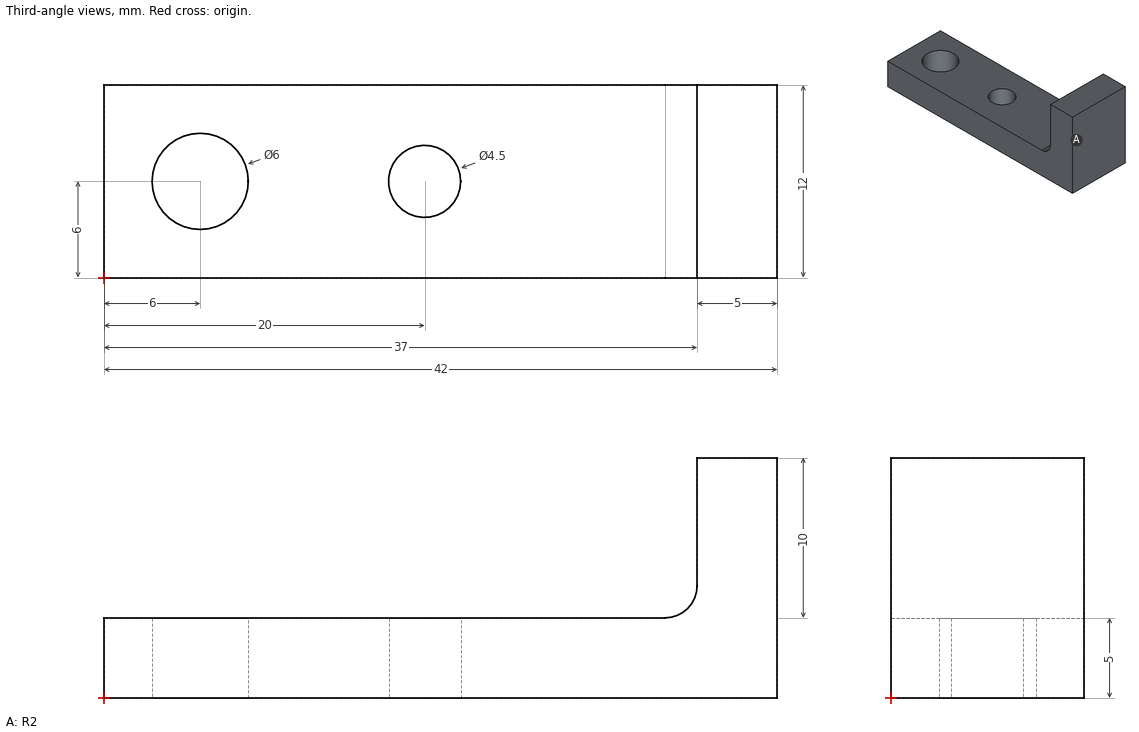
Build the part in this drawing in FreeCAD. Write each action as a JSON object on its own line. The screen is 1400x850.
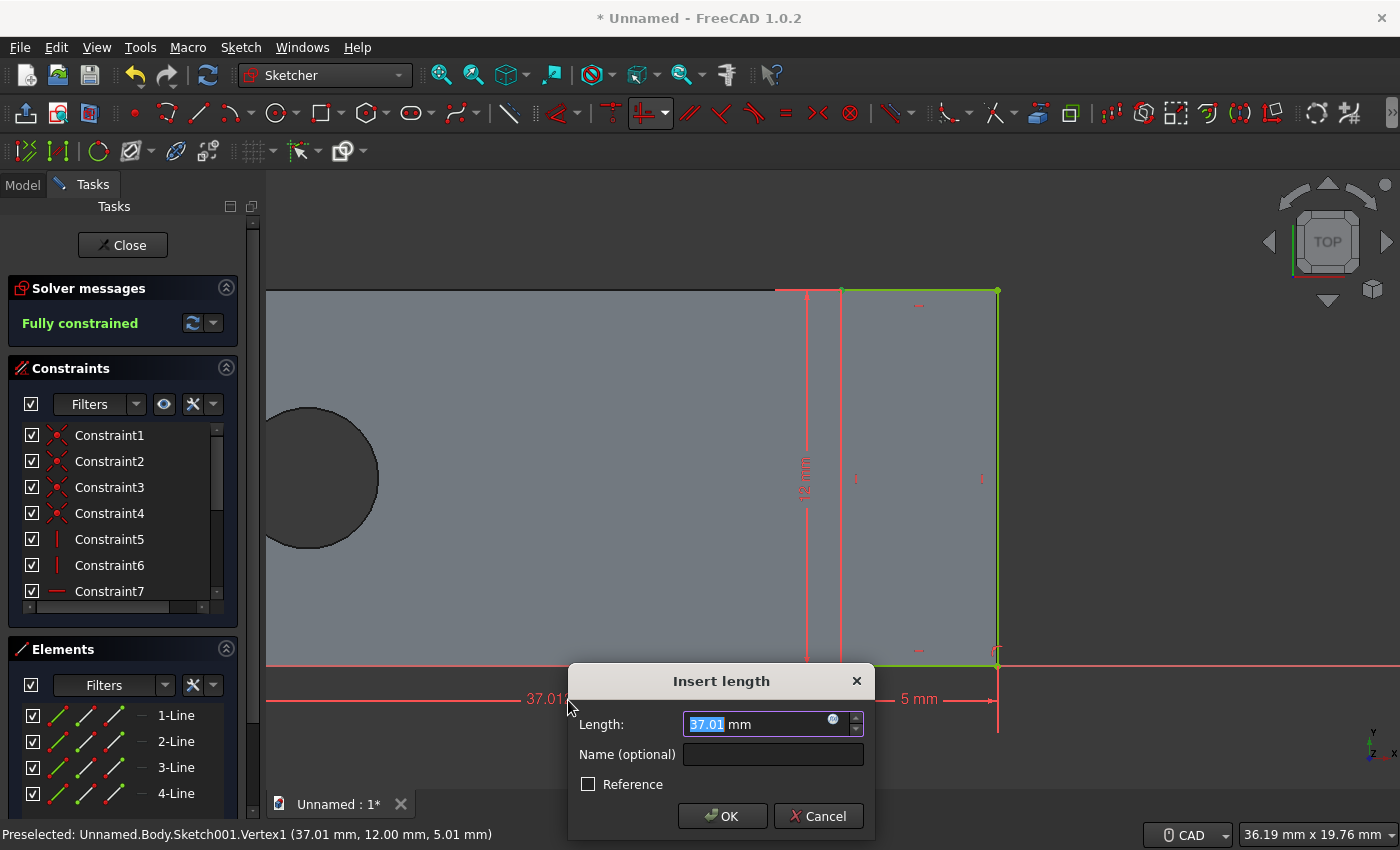
{"action": "type", "text": "37"}
{"action": "key", "text": "Return"}
{"action": "key", "text": "Escape"}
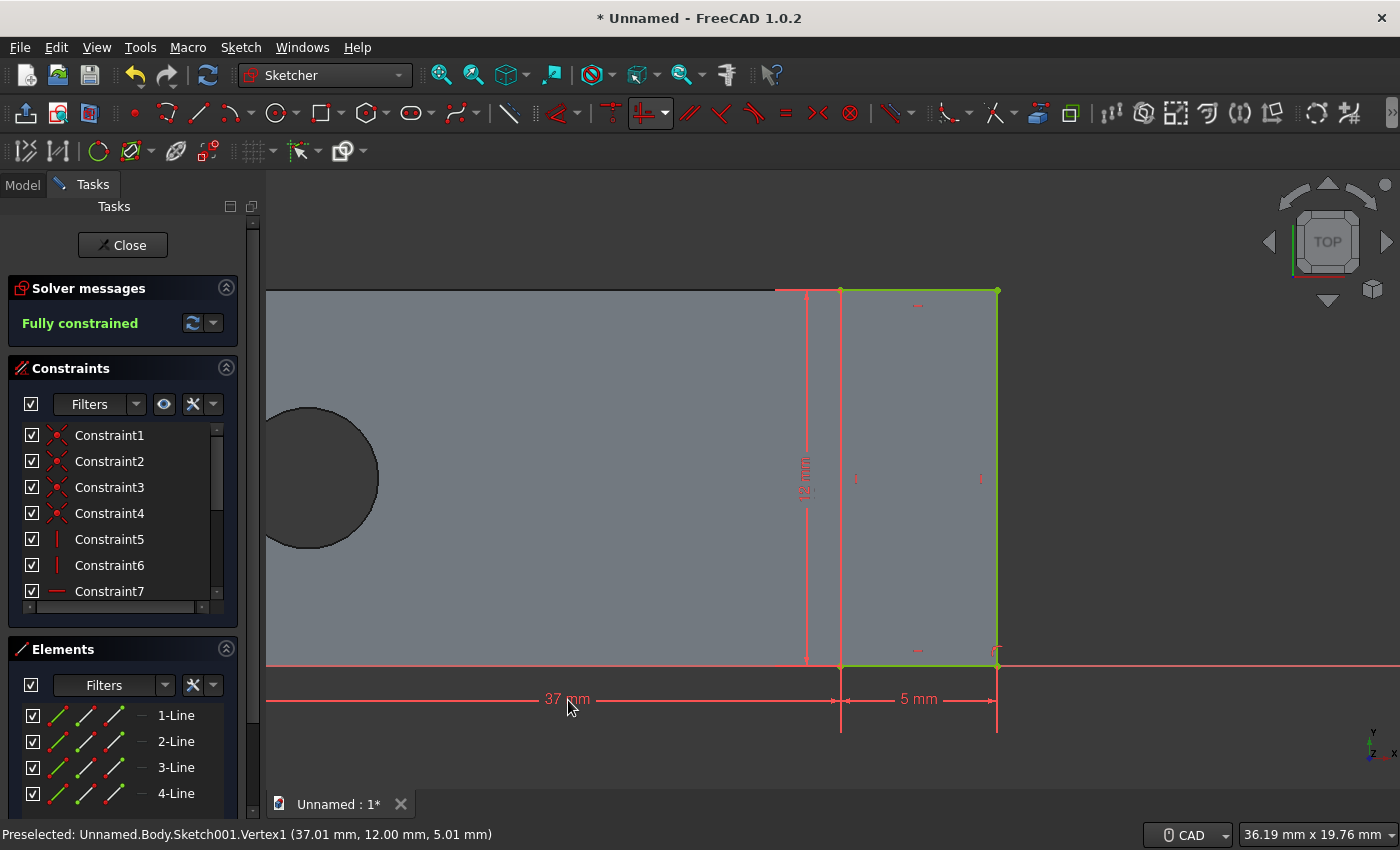
{"action": "left_click", "coordinate": [123, 245]}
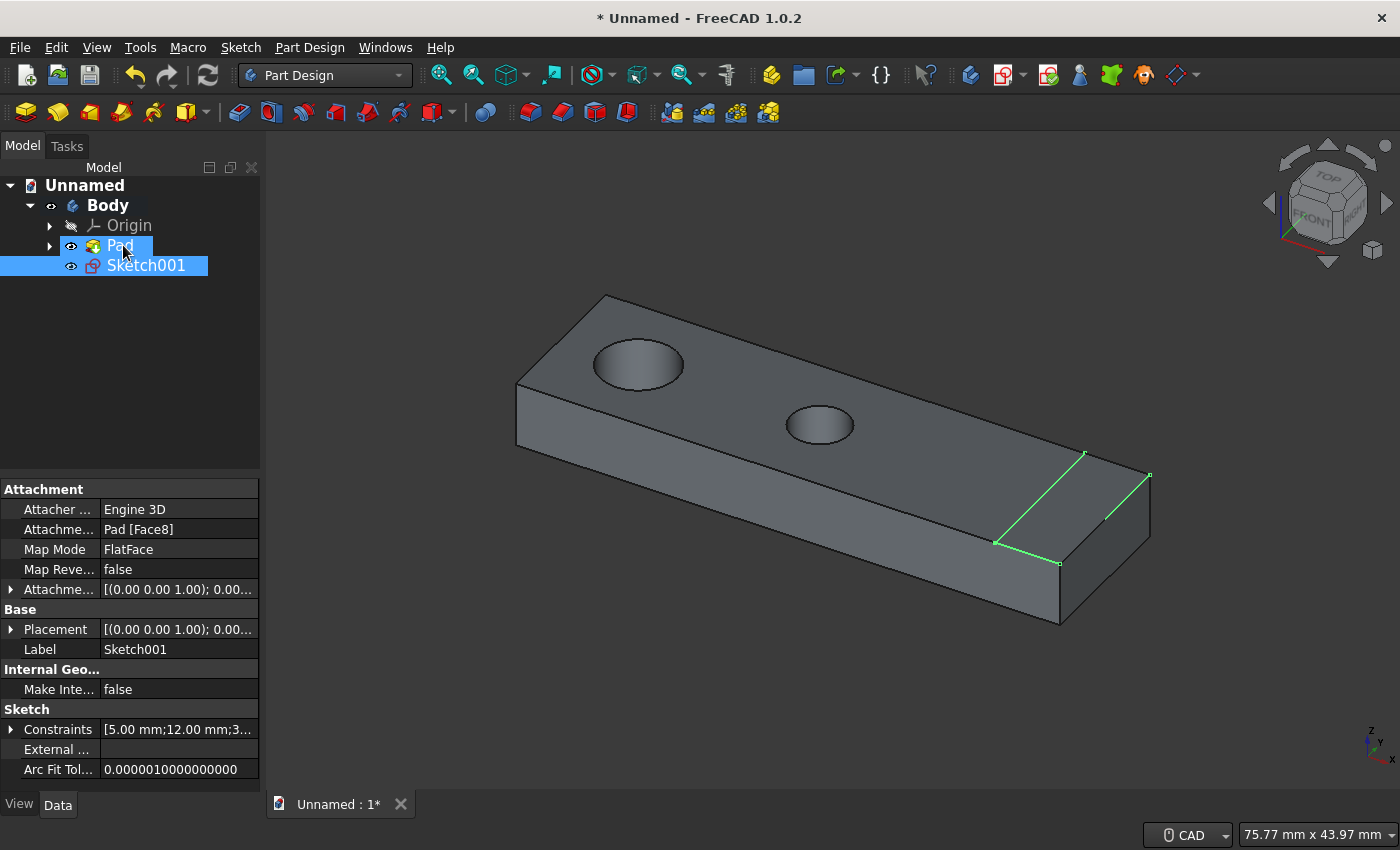
{"action": "left_click", "coordinate": [26, 112]}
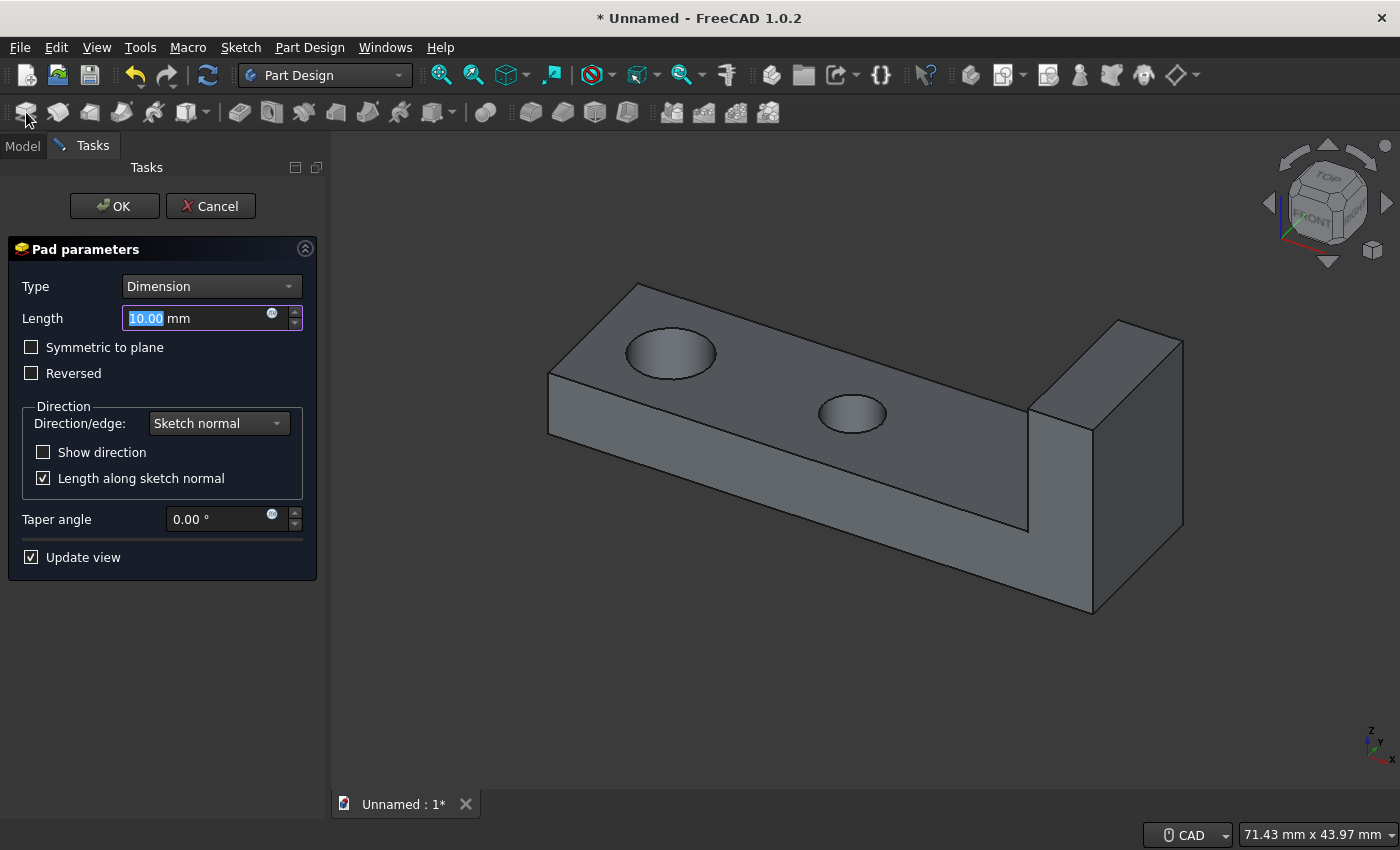
{"action": "type", "text": "10"}
{"action": "key", "text": "Tab"}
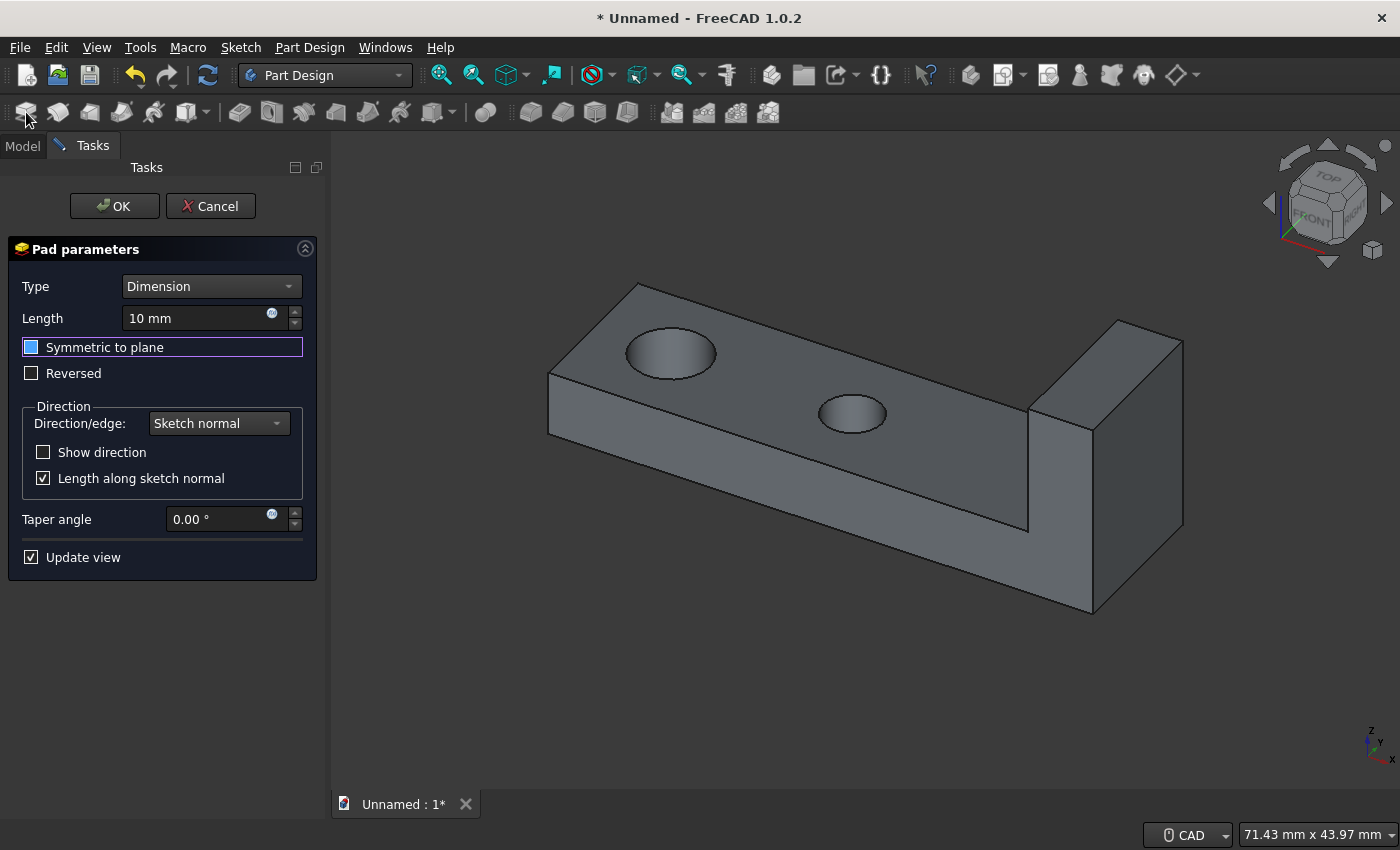
{"action": "left_click", "coordinate": [115, 206]}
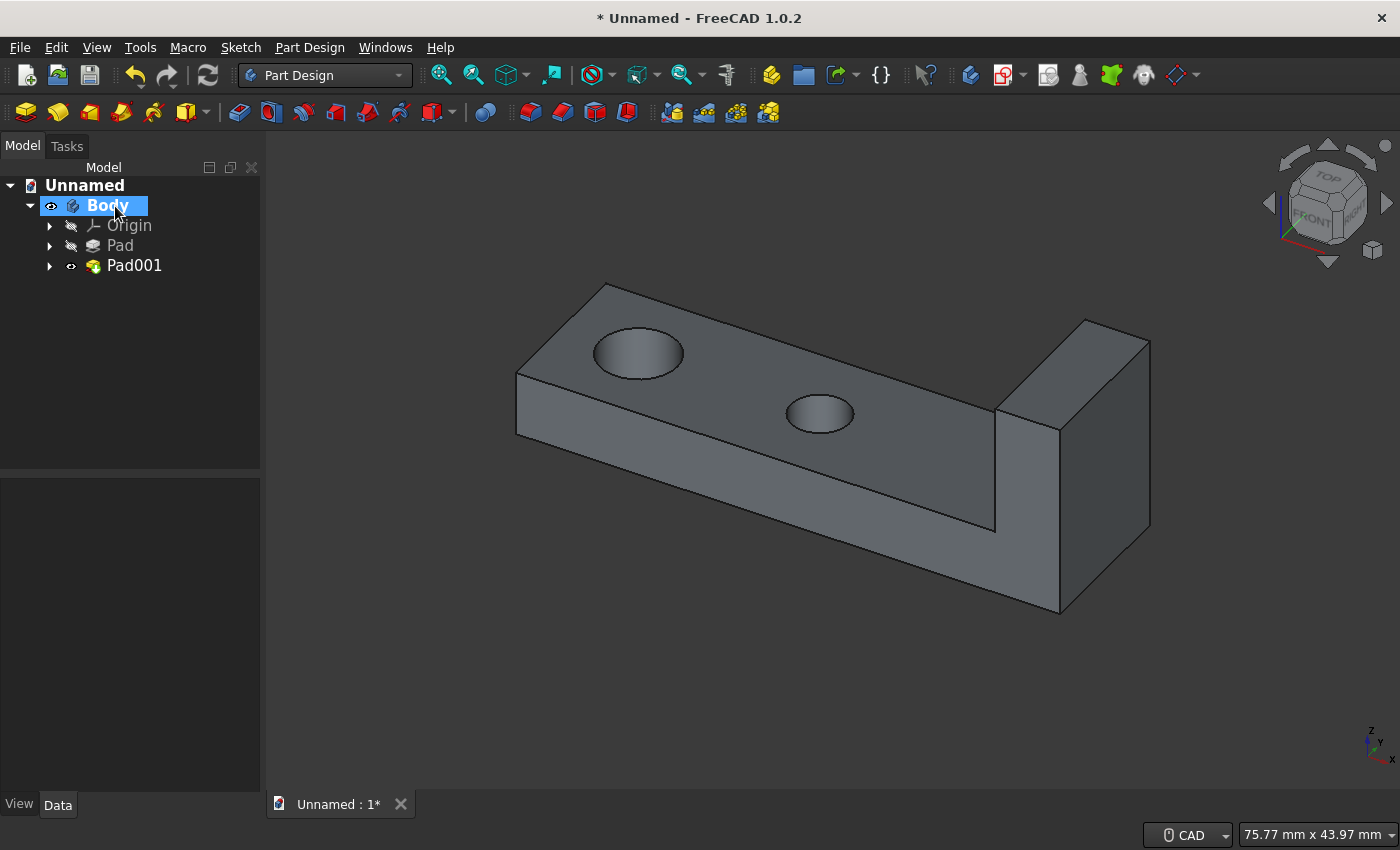
{"action": "key", "text": "0"}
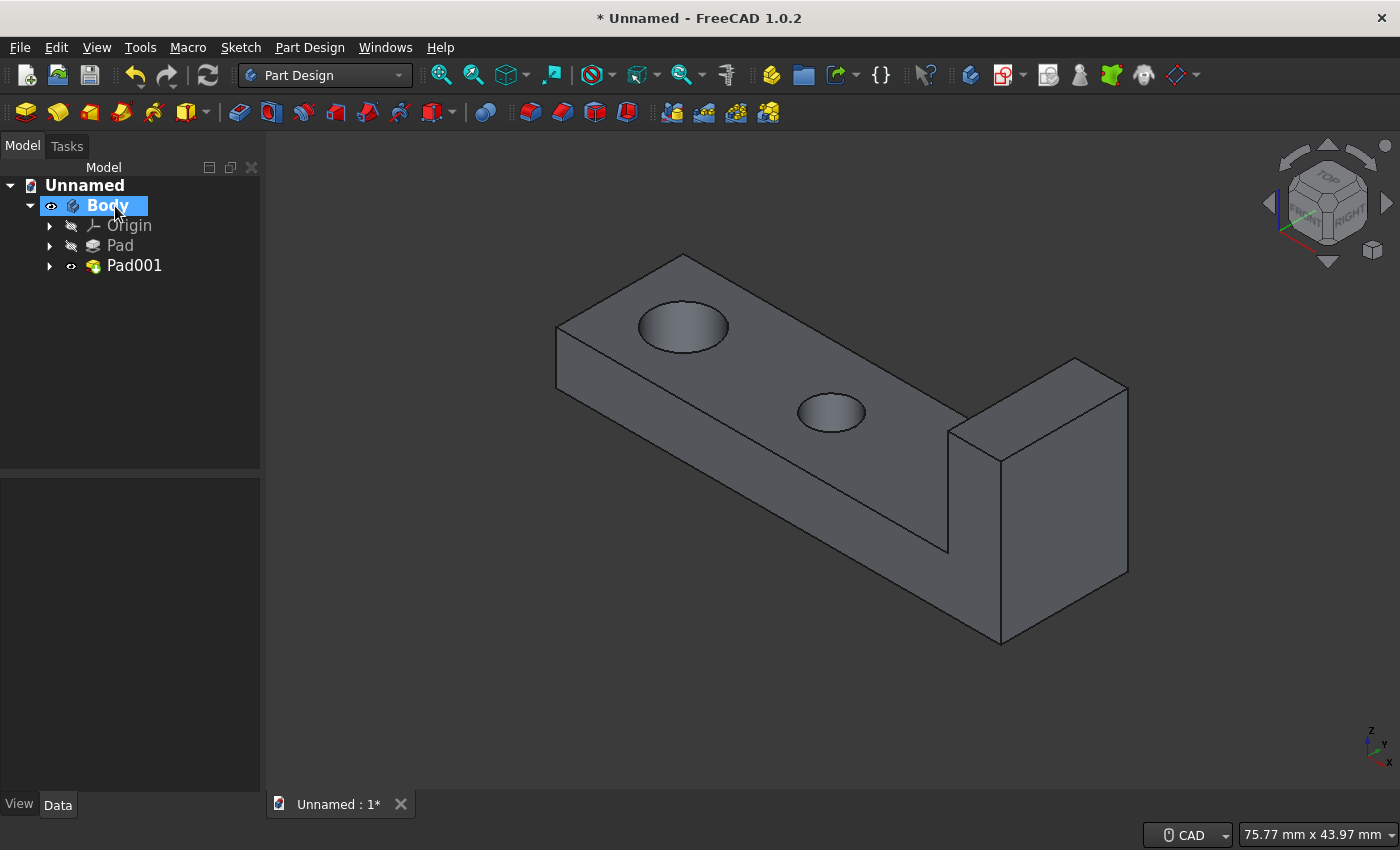
{"action": "key", "text": "2"}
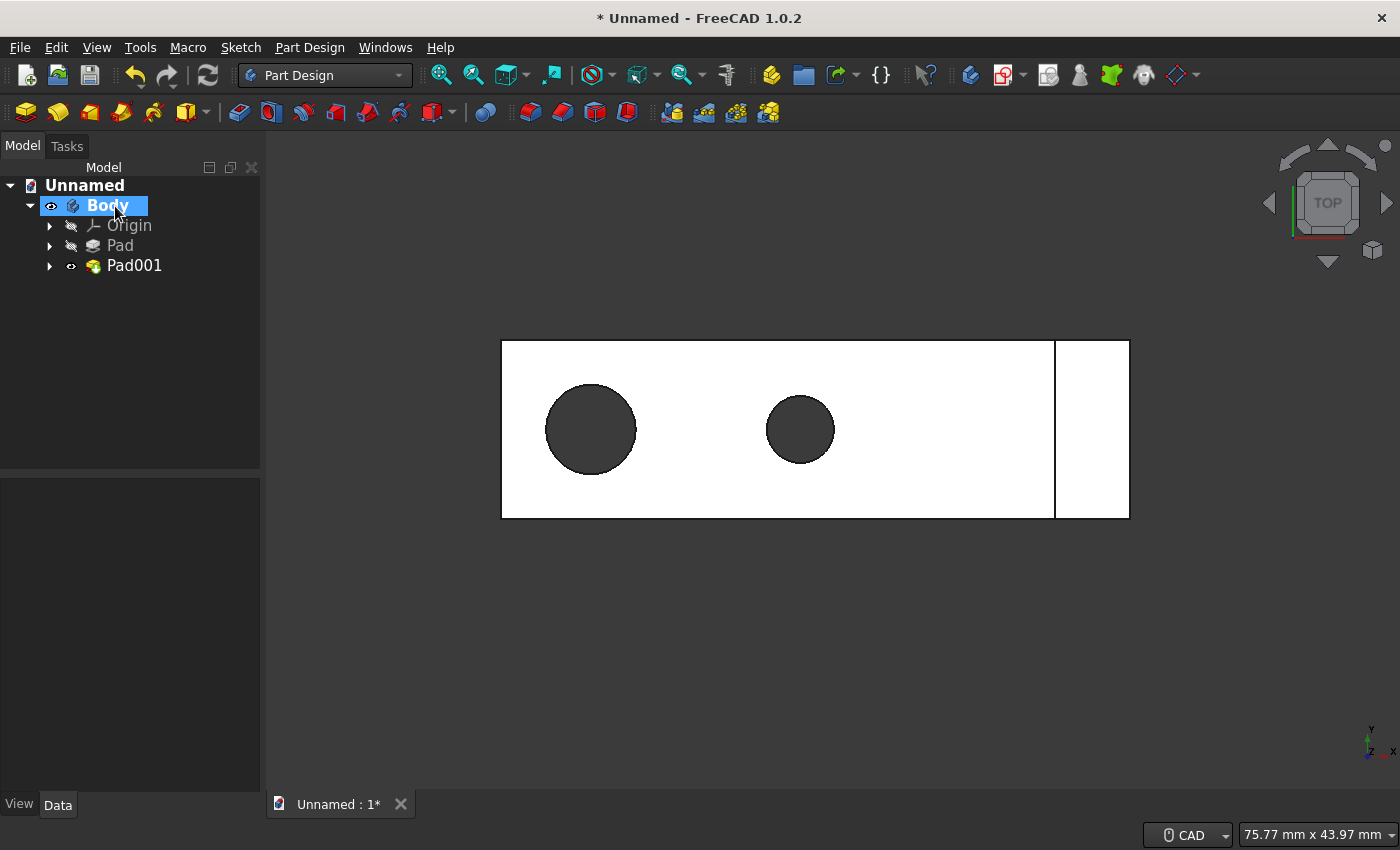
{"action": "key", "text": "1"}